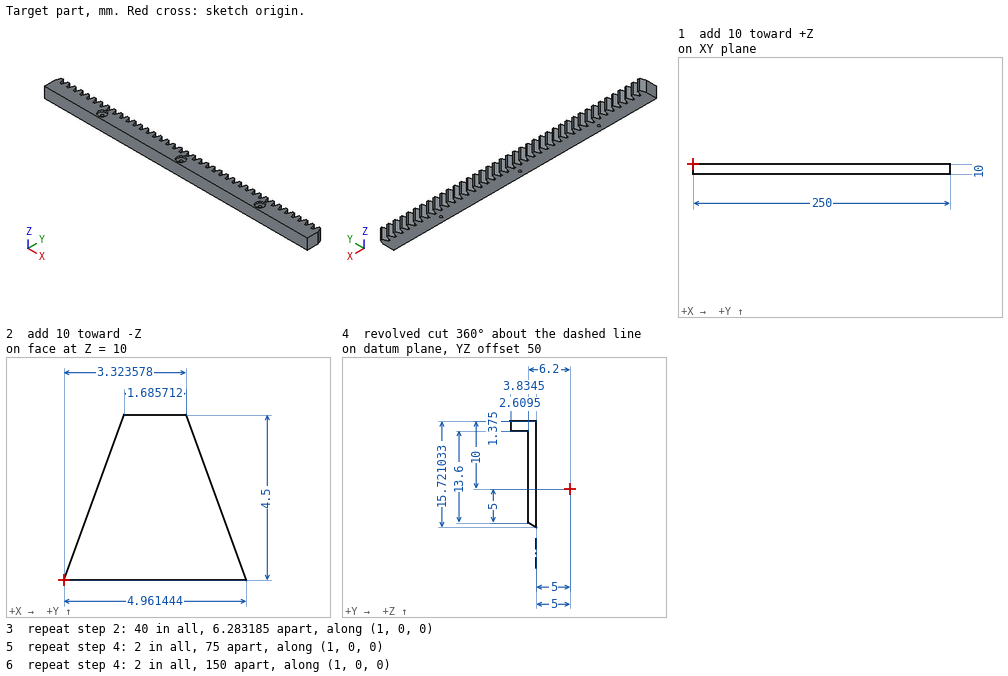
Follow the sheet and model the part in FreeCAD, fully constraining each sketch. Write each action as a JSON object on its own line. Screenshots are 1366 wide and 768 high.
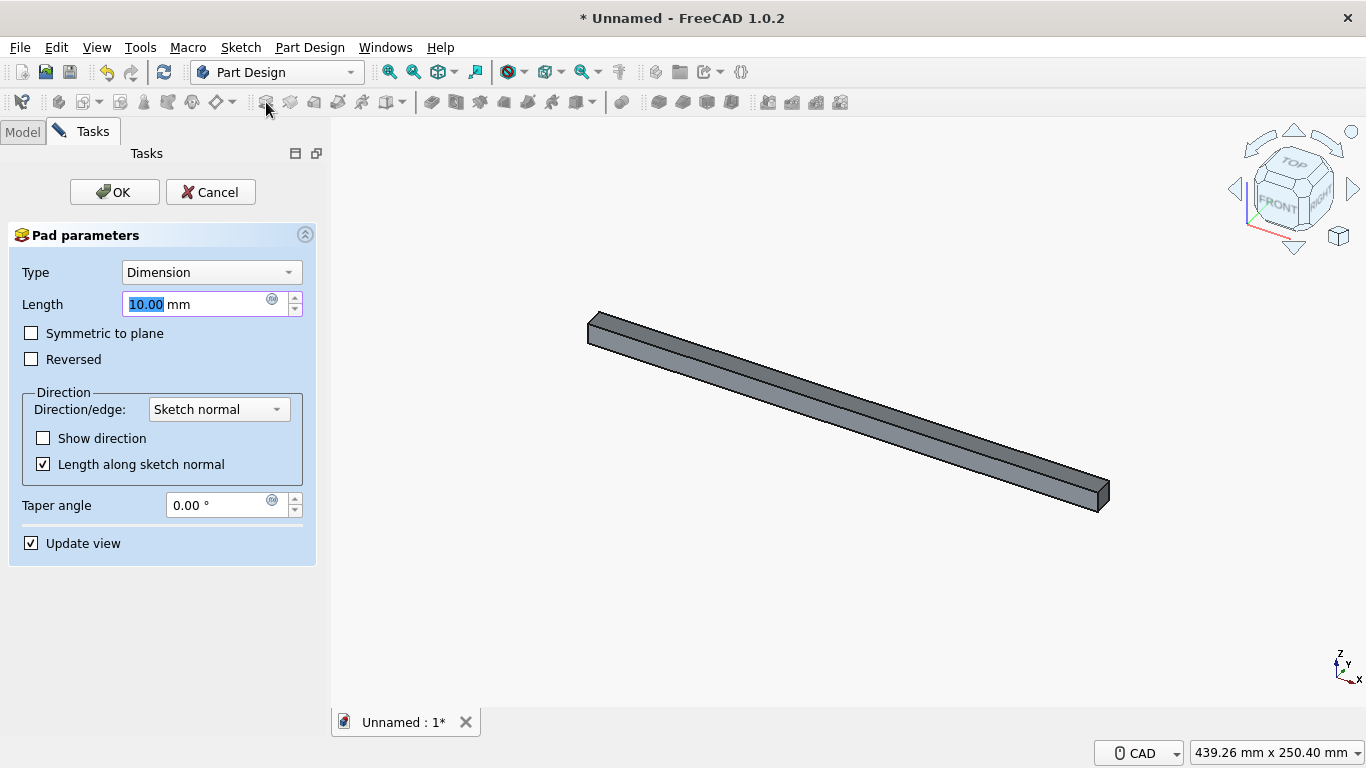
{"action": "type", "text": "10"}
{"action": "key", "text": "Tab"}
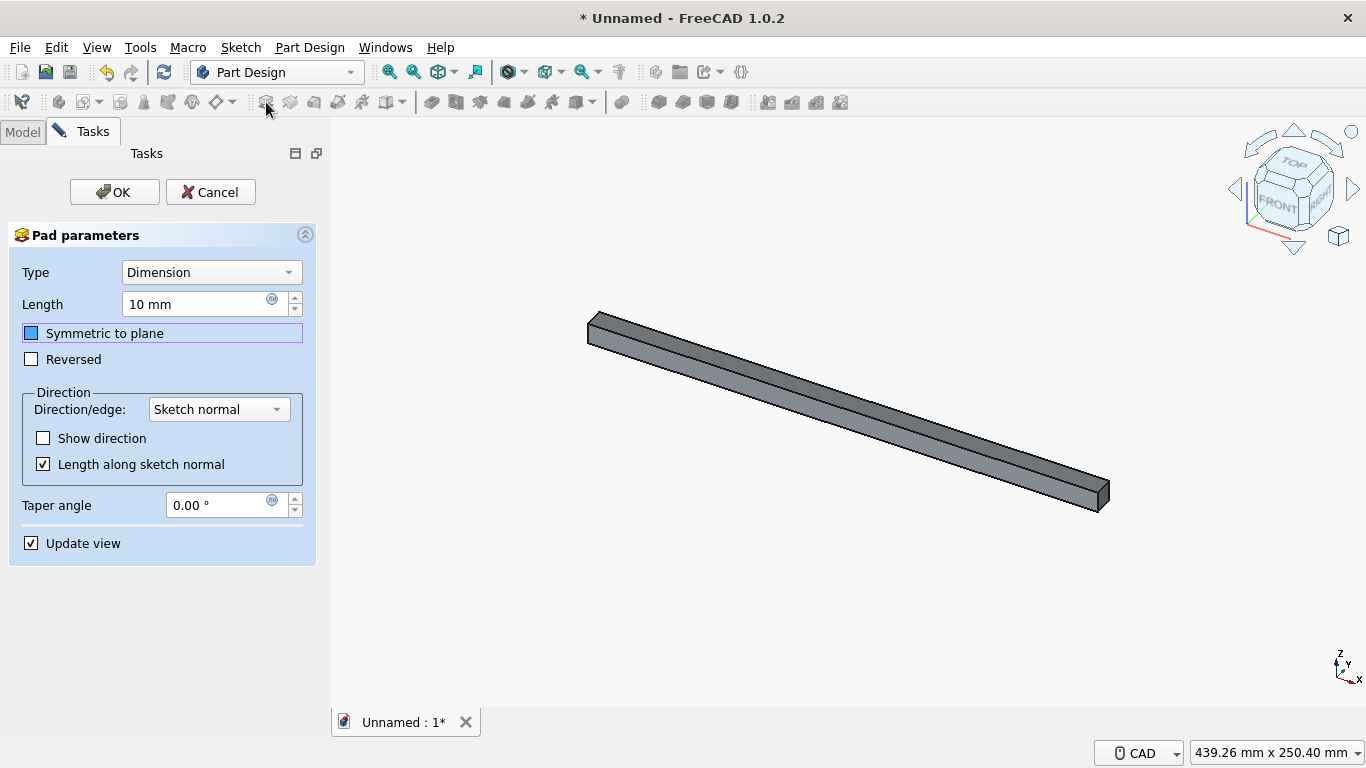
{"action": "left_click", "coordinate": [30, 359]}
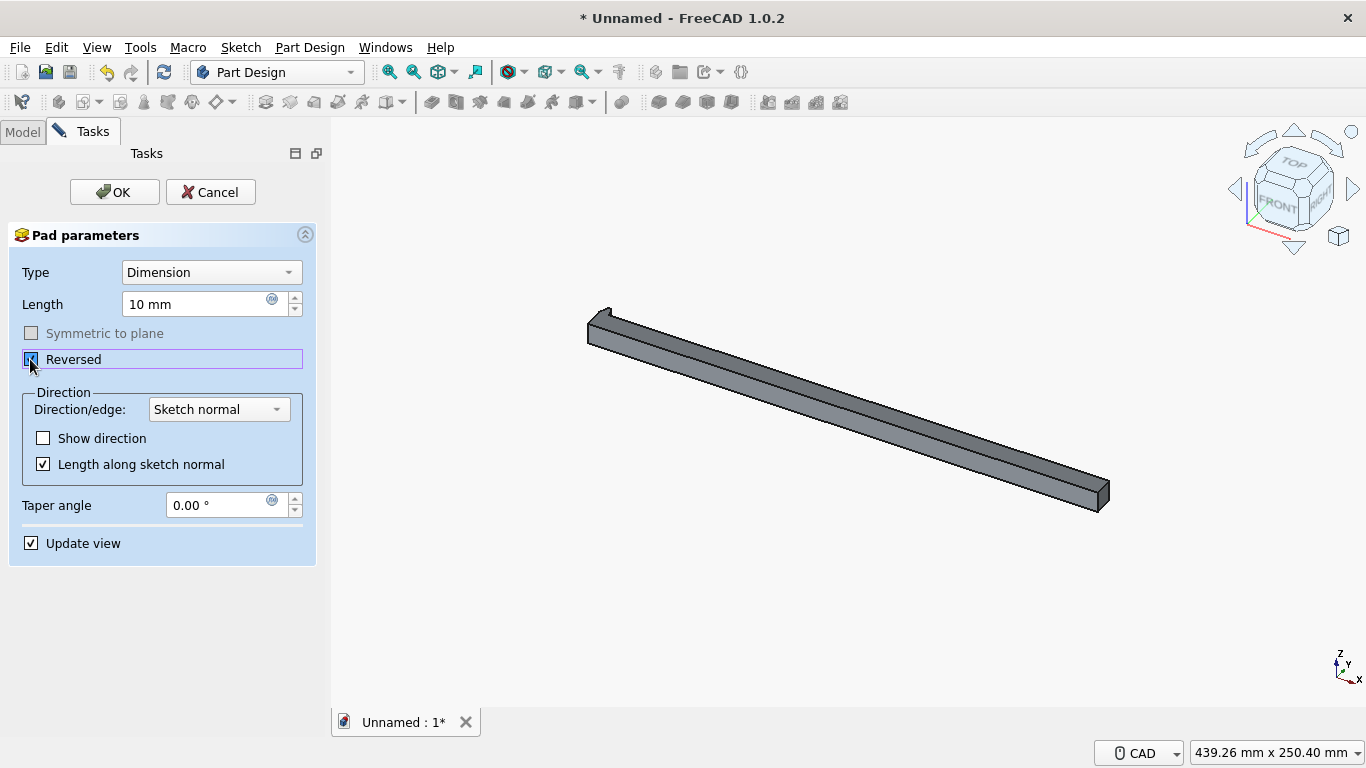
{"action": "left_click", "coordinate": [115, 192]}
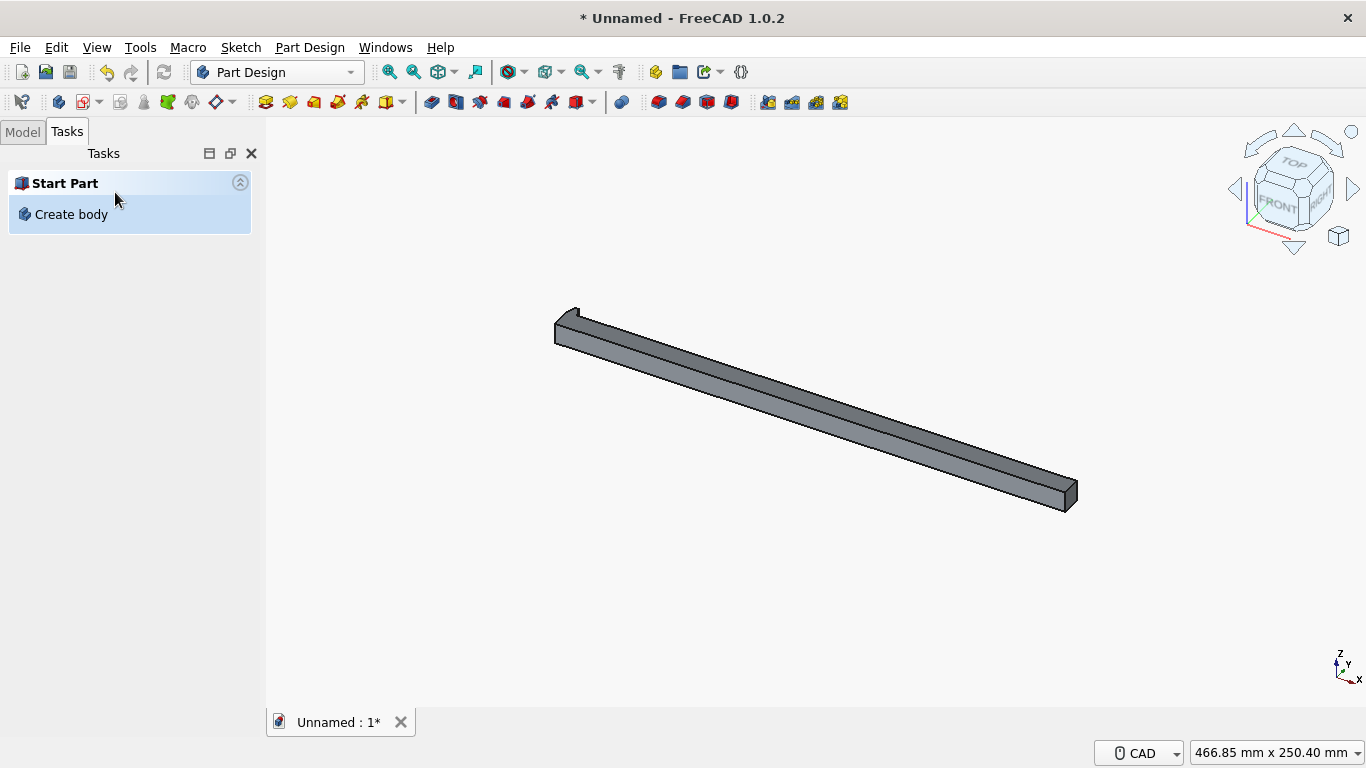
{"action": "left_click", "coordinate": [23, 131]}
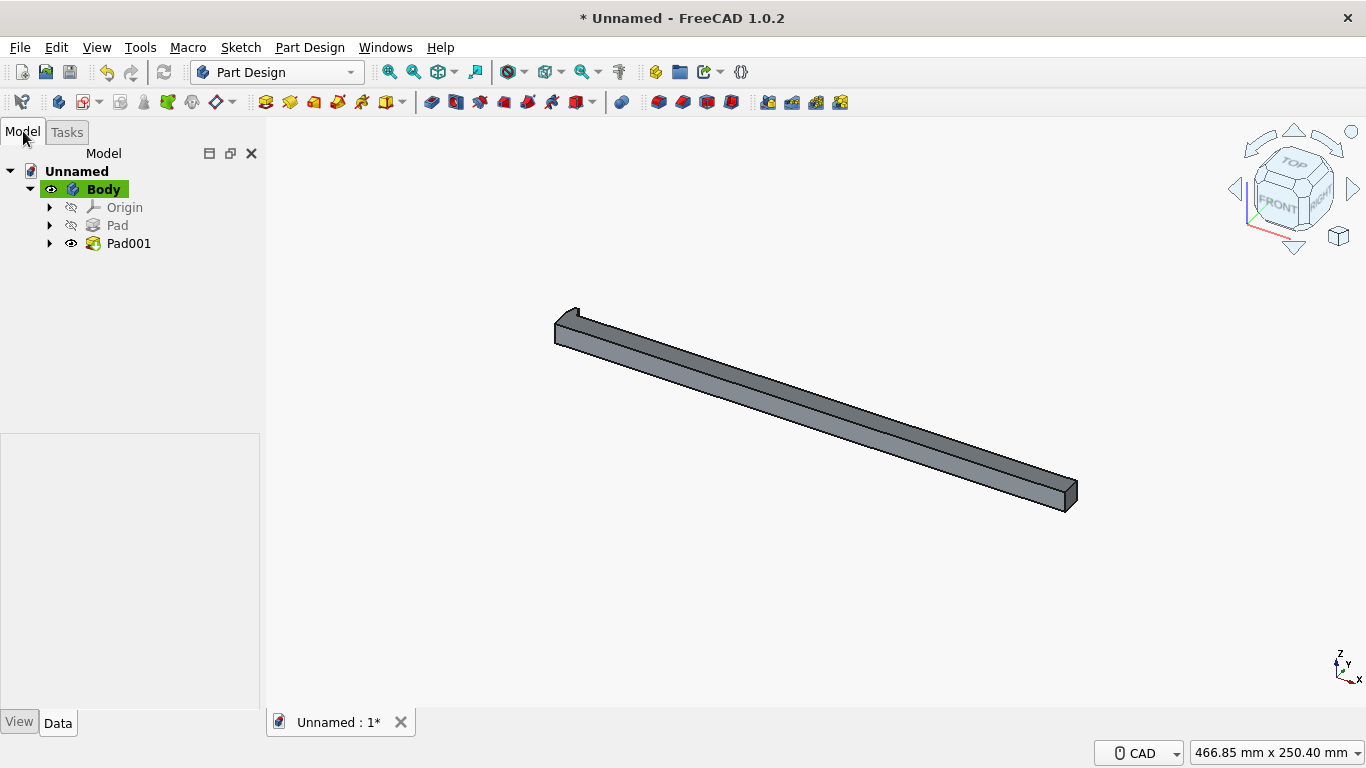
{"action": "left_click", "coordinate": [116, 243]}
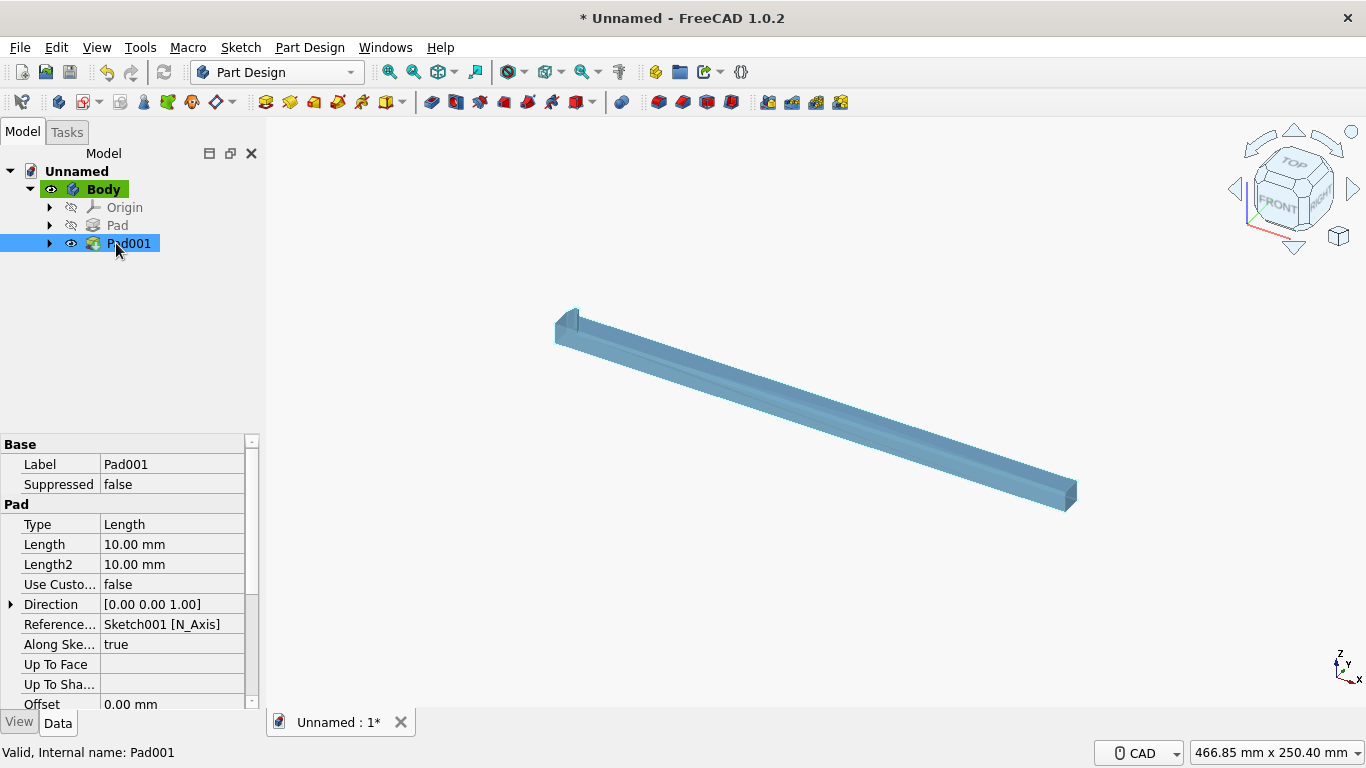
{"action": "left_click", "coordinate": [792, 102]}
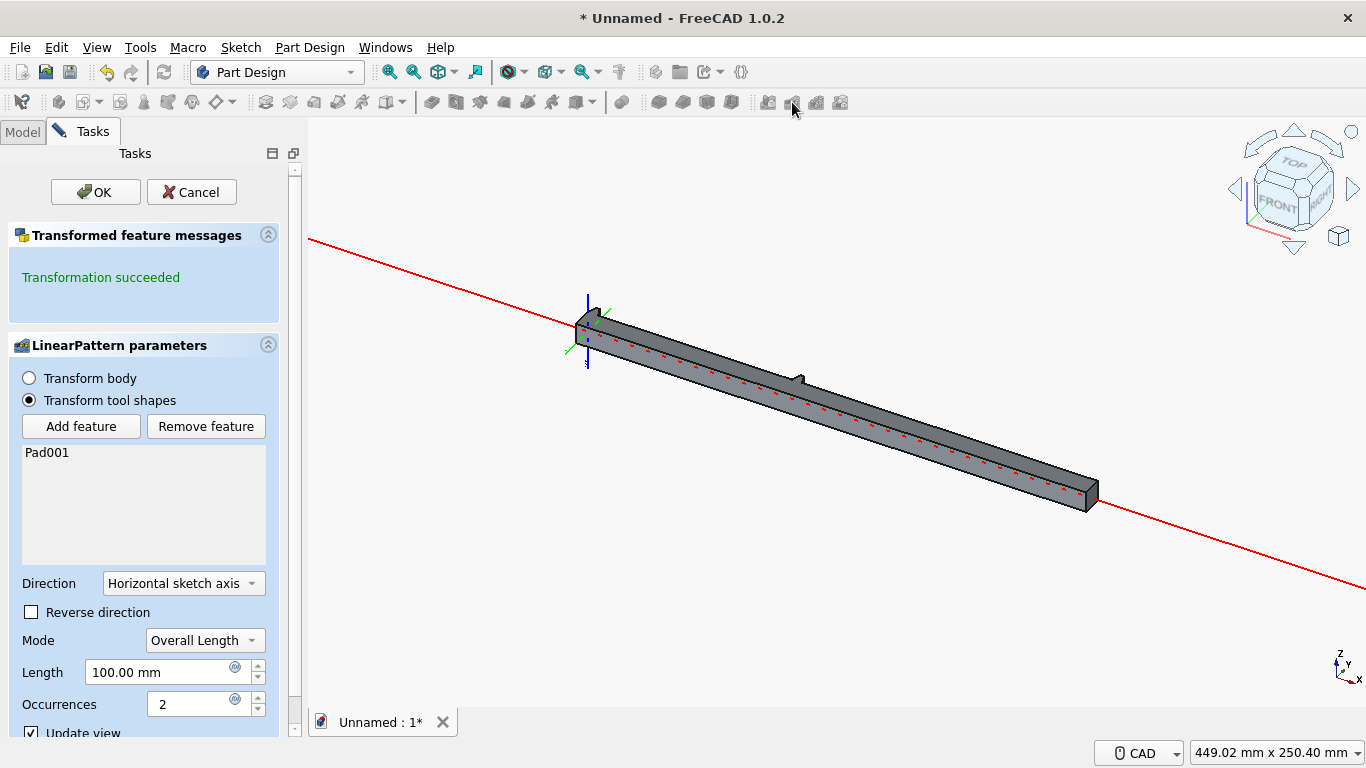
{"action": "left_click", "coordinate": [184, 584]}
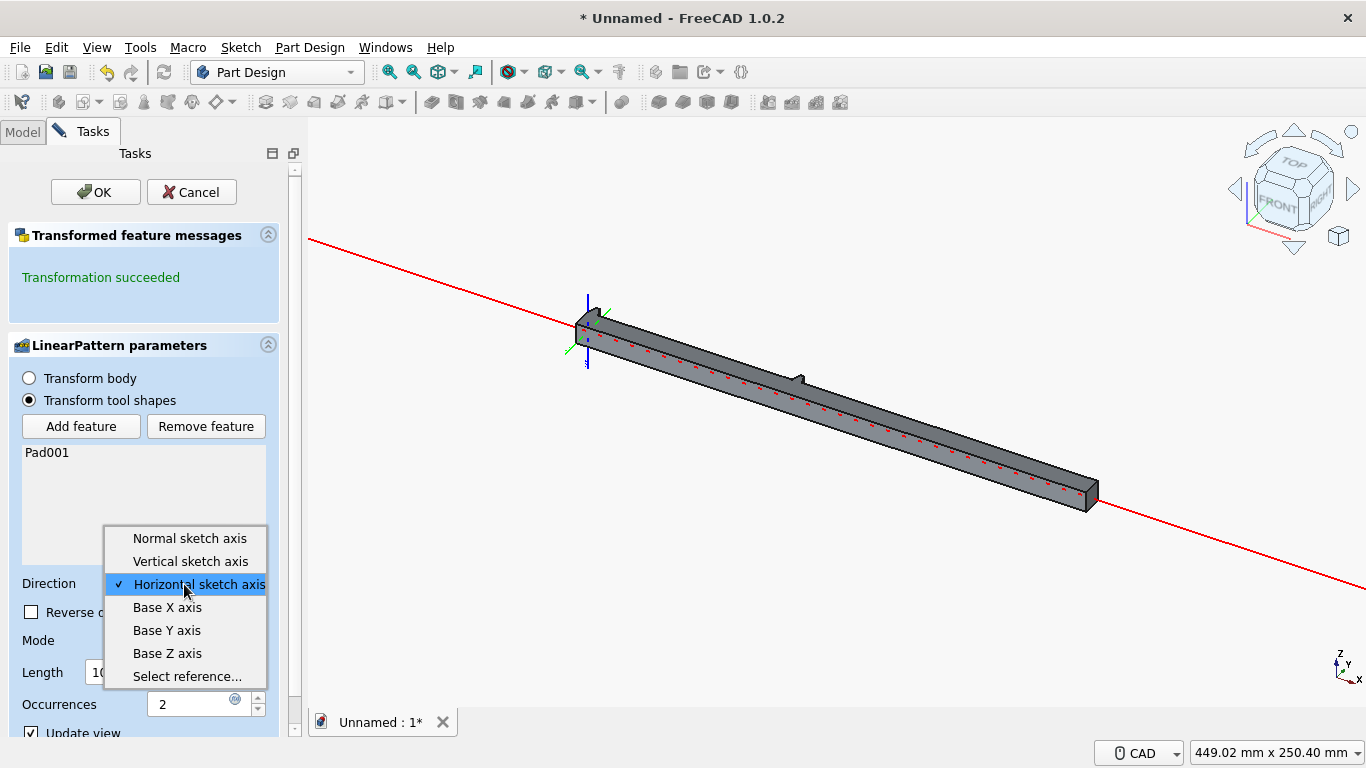
{"action": "left_click", "coordinate": [184, 608]}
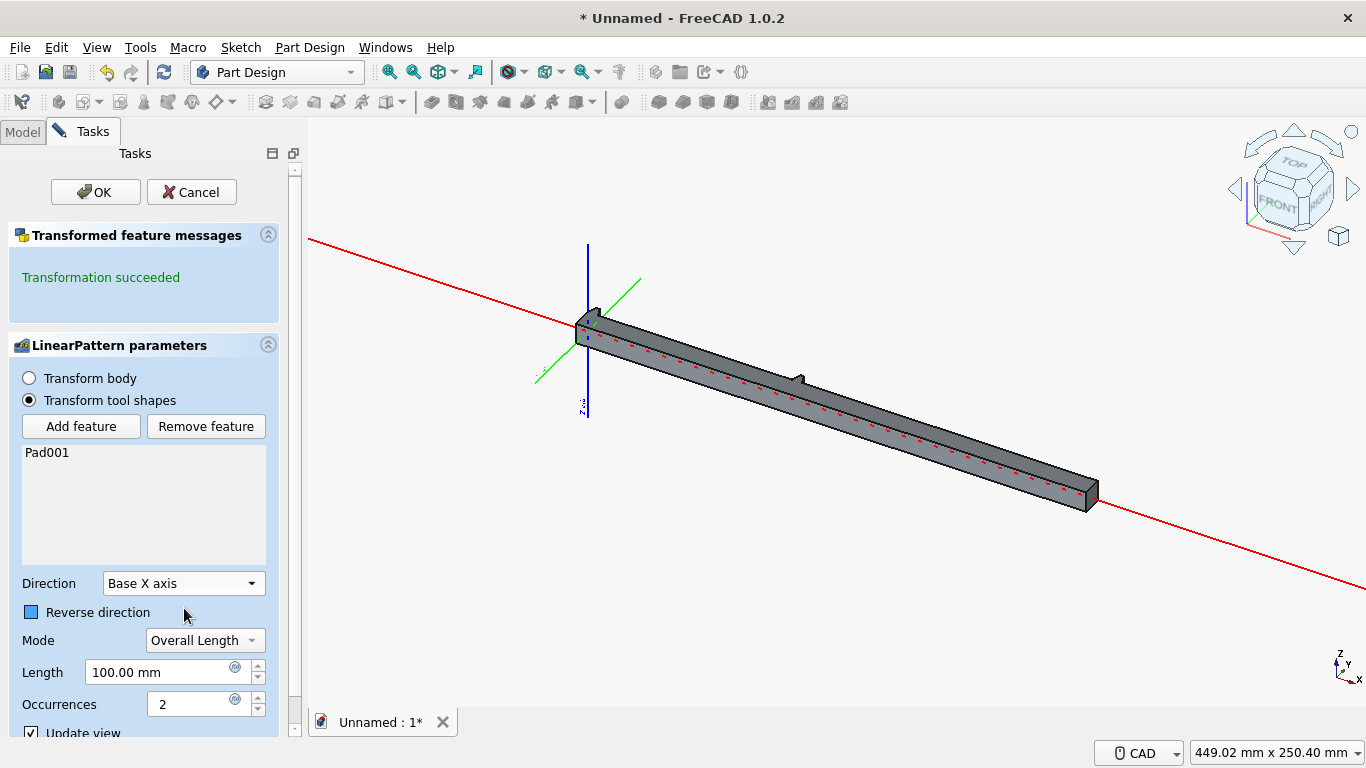
{"action": "left_click", "coordinate": [206, 640]}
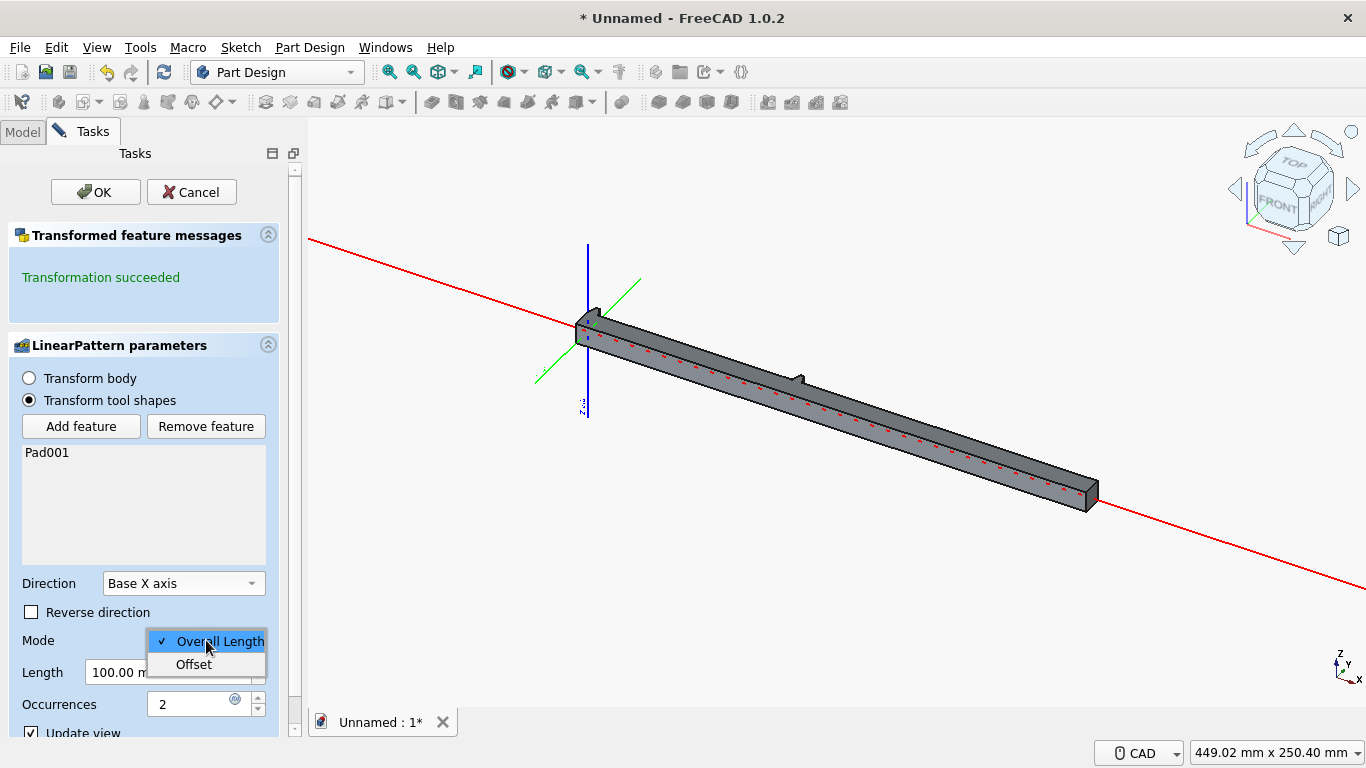
{"action": "left_click", "coordinate": [206, 664]}